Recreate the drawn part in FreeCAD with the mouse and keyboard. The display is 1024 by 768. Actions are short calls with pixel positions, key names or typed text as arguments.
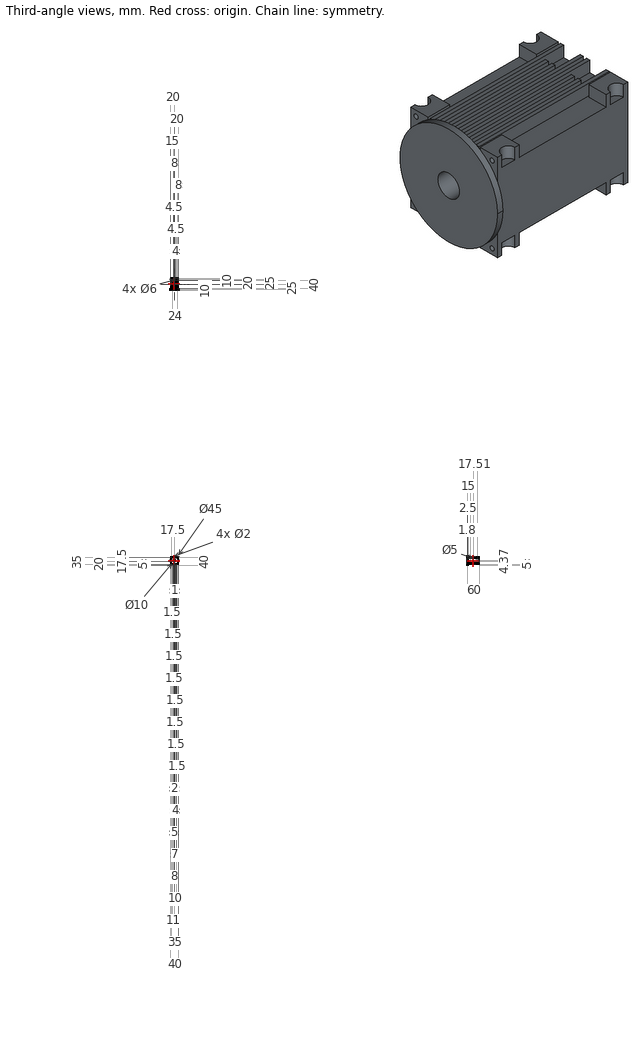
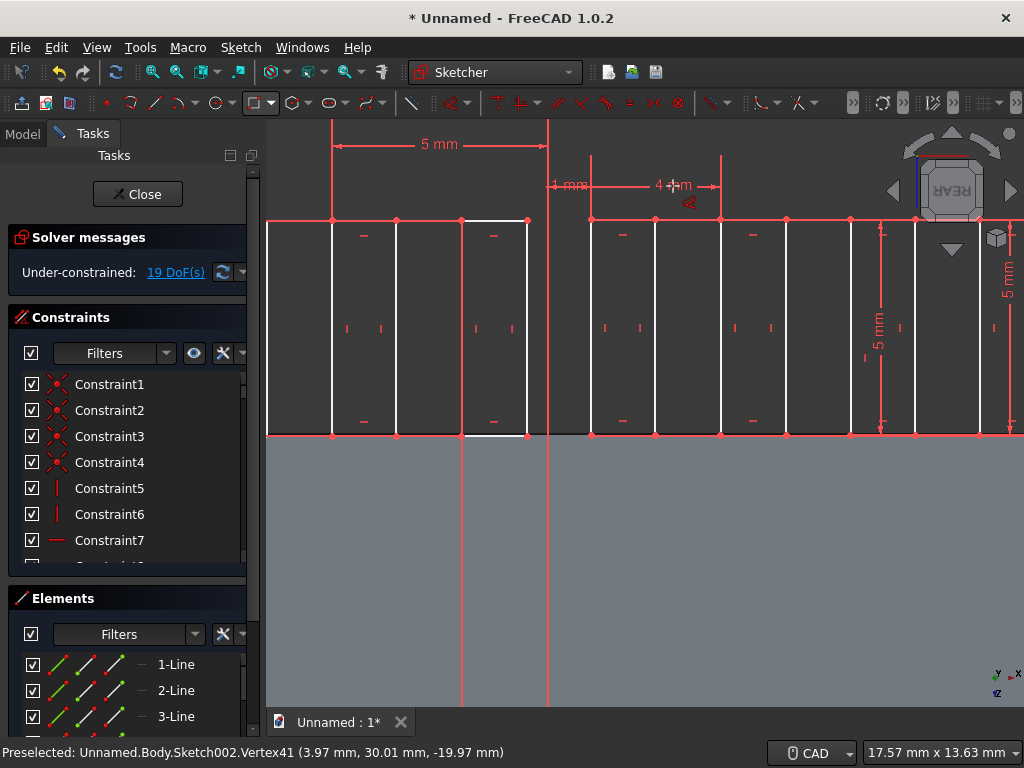
click(851, 220)
click(769, 186)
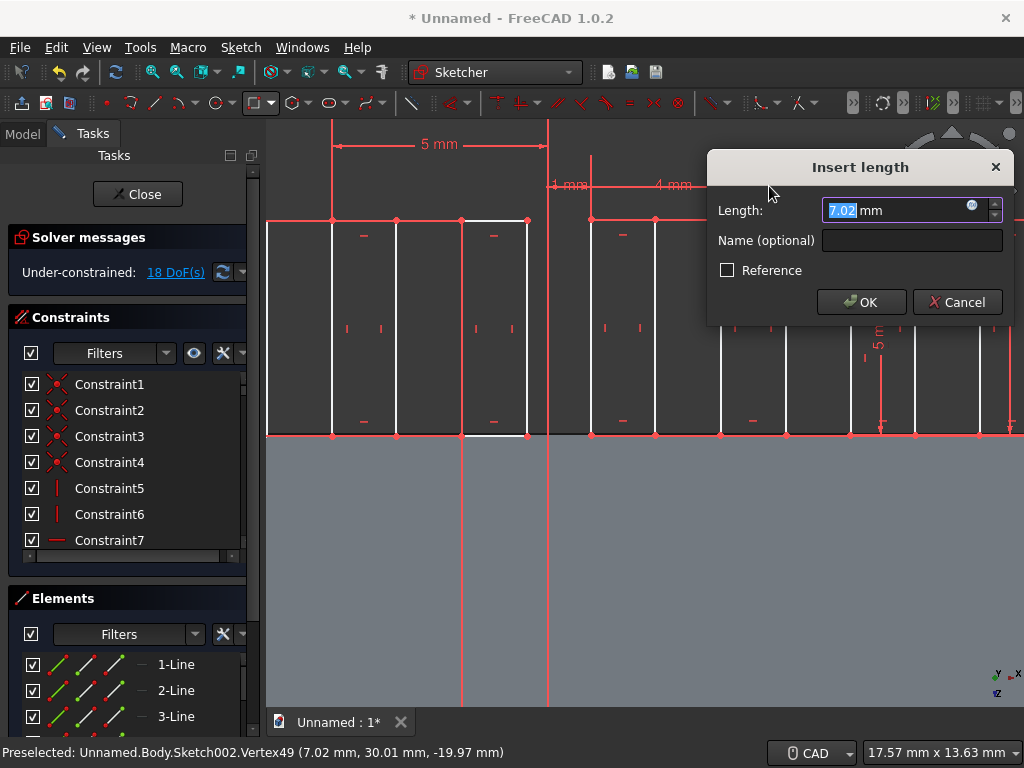
text(7)
key(Return)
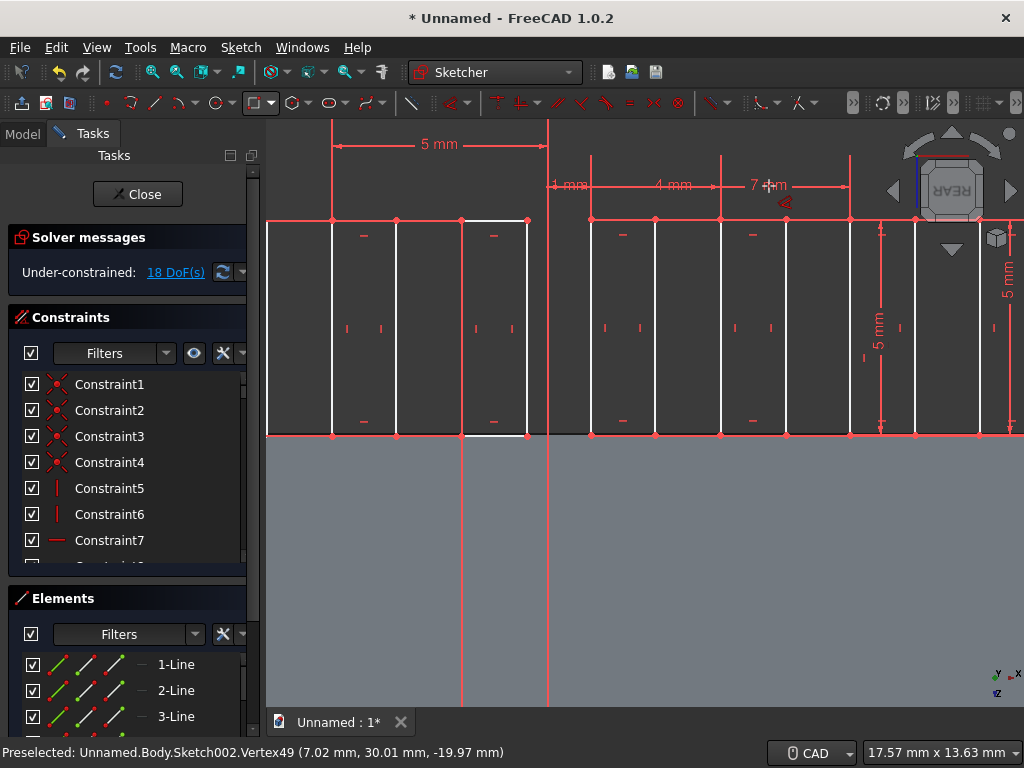
scroll(591, 220, down, 4)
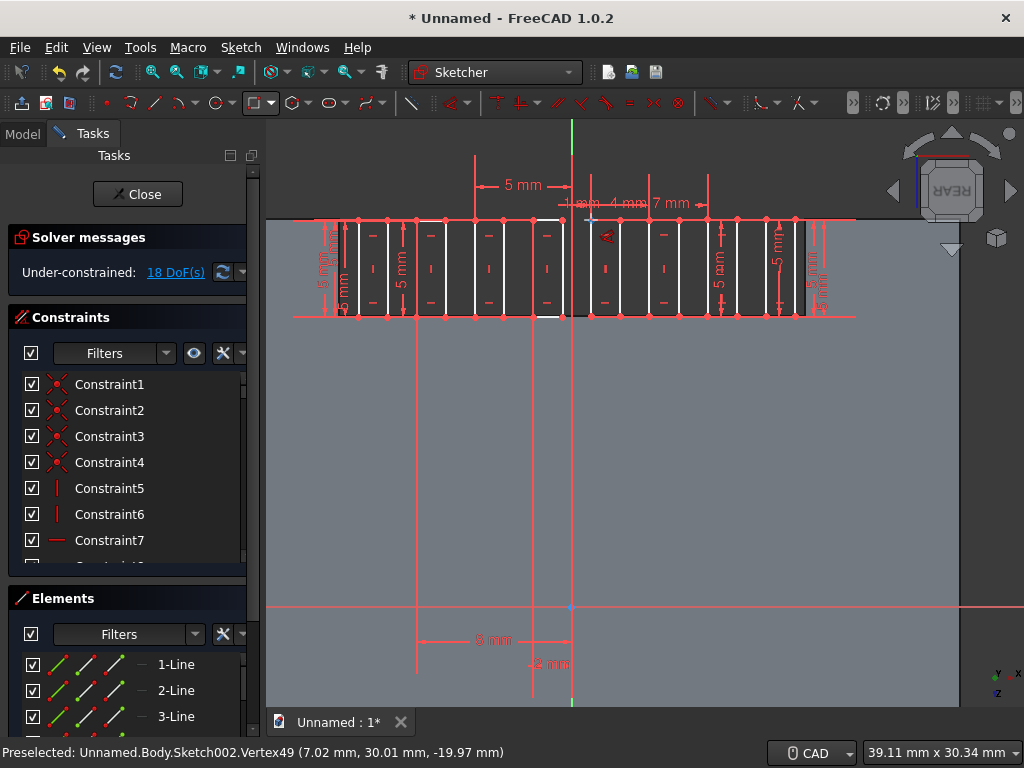
scroll(368, 317, up, 3)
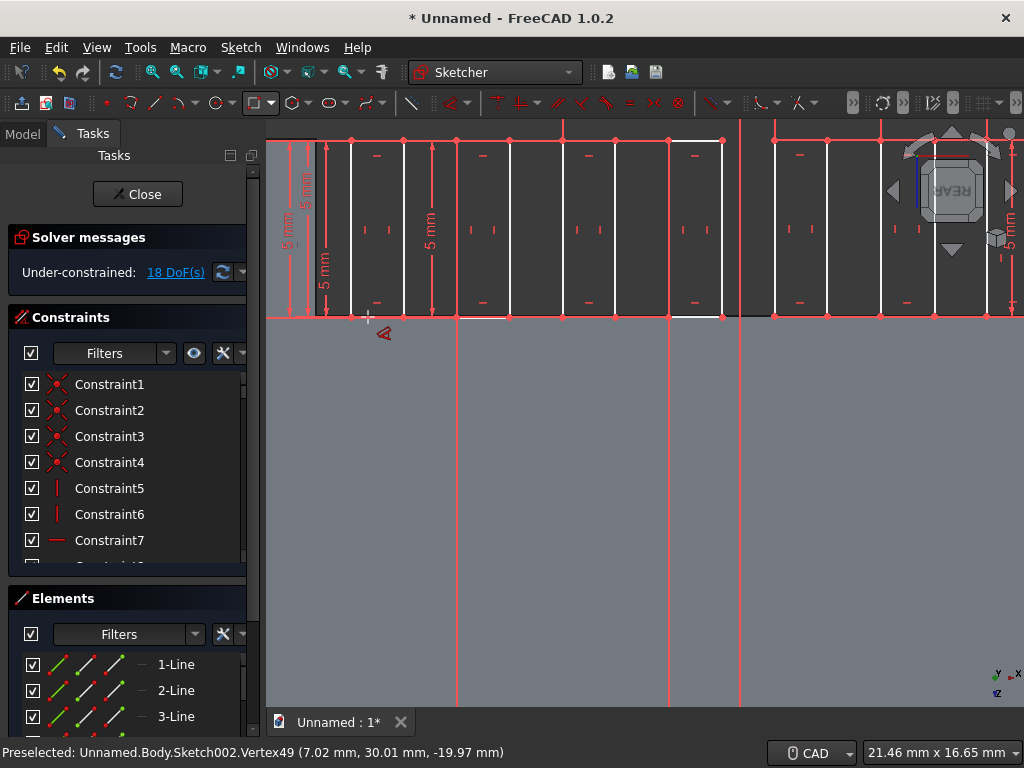
click(367, 318)
click(378, 352)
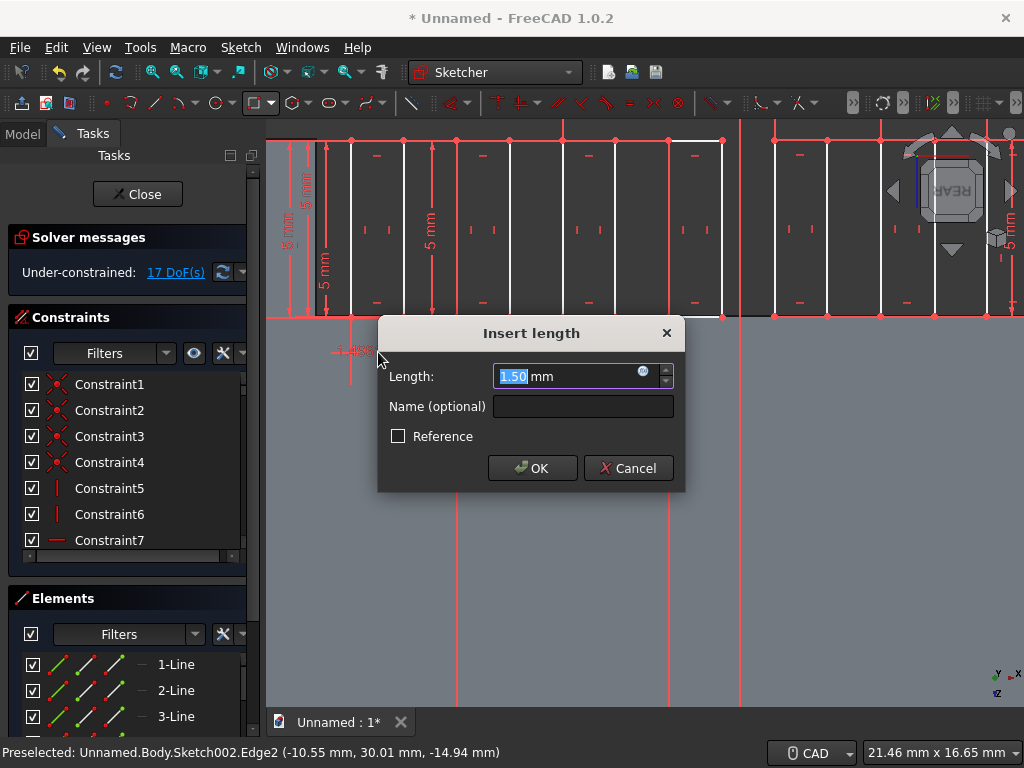
text(1.5)
key(Return)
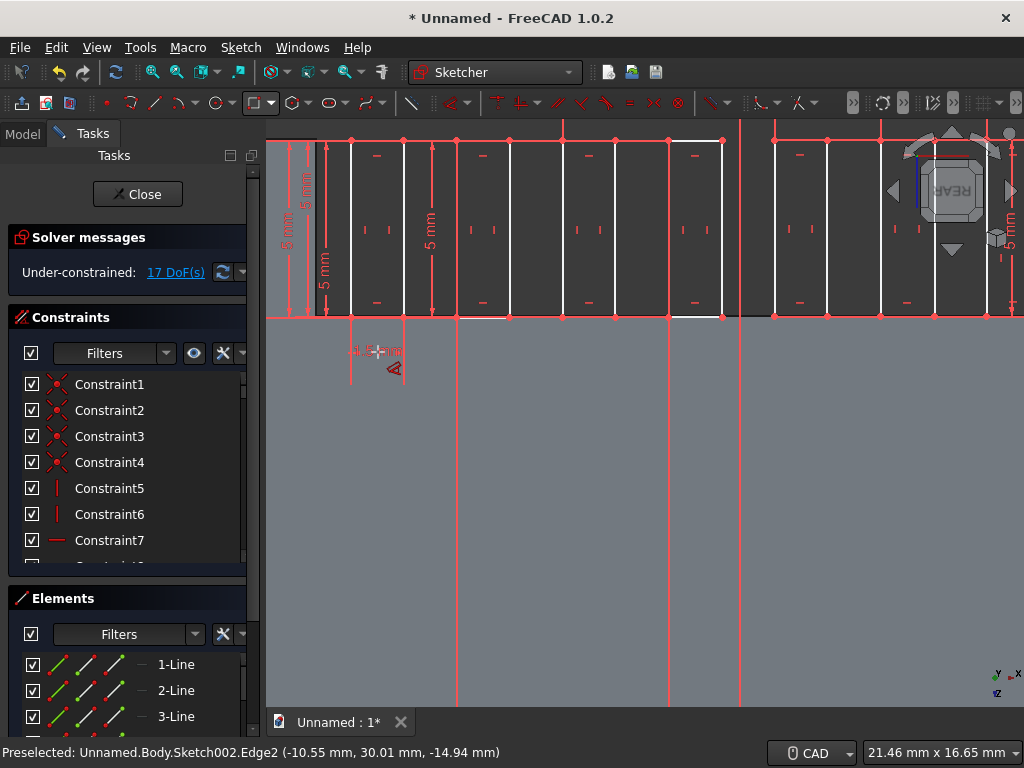
click(473, 318)
click(483, 284)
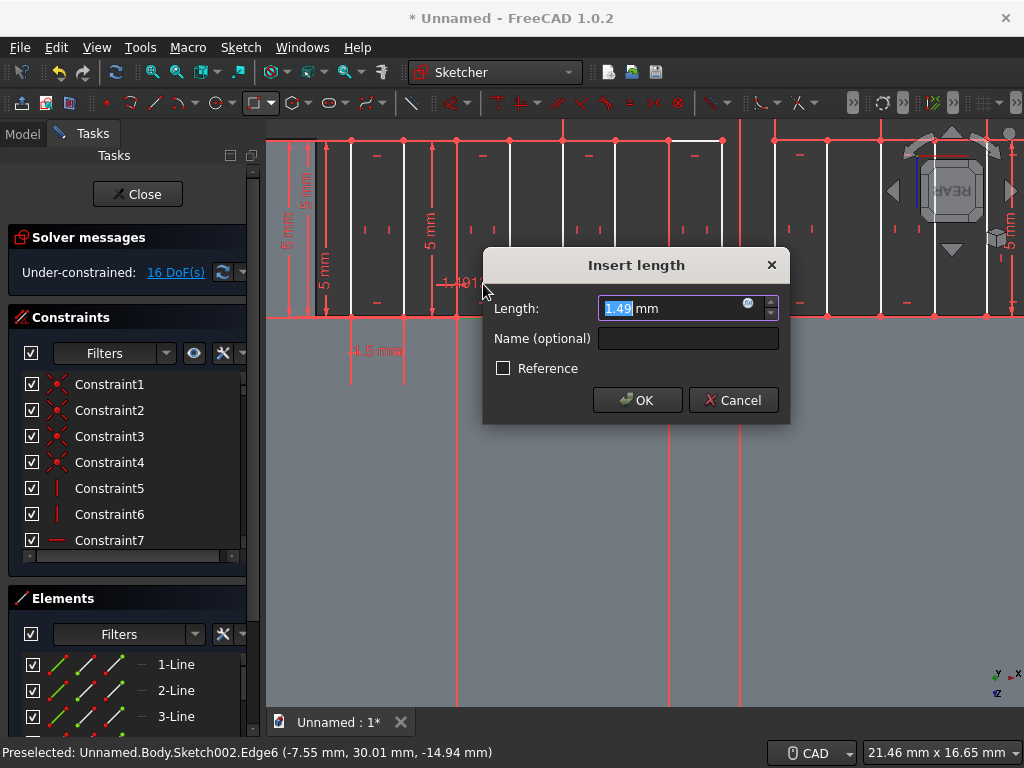
text(1.5)
key(Return)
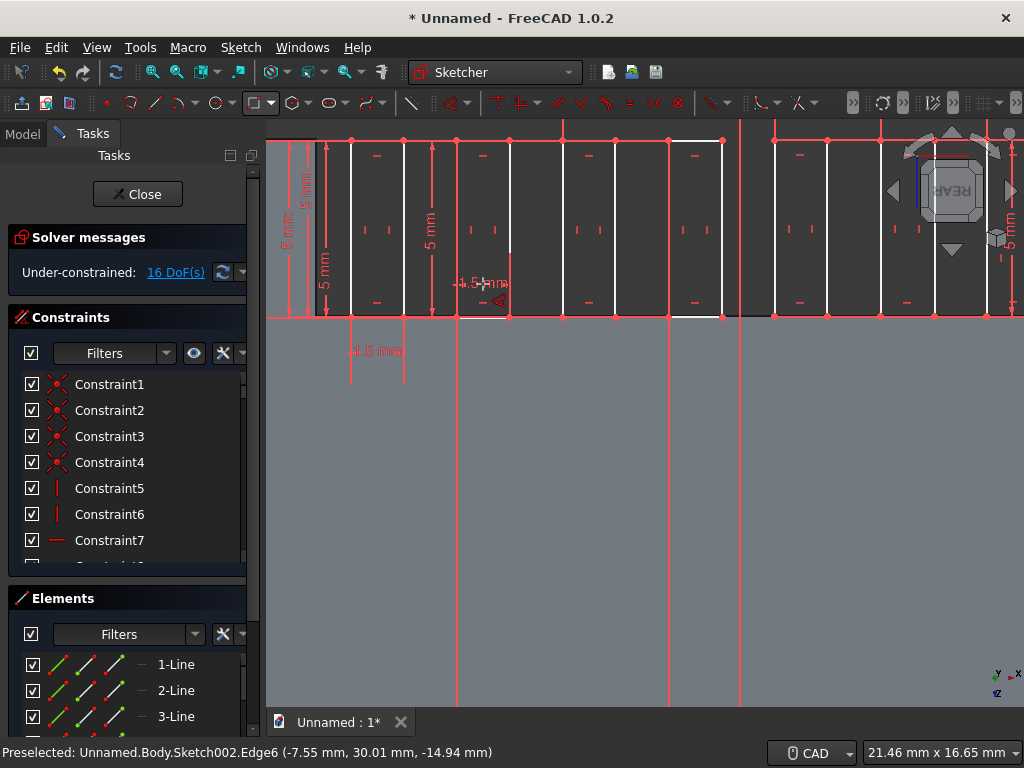
click(579, 317)
click(589, 283)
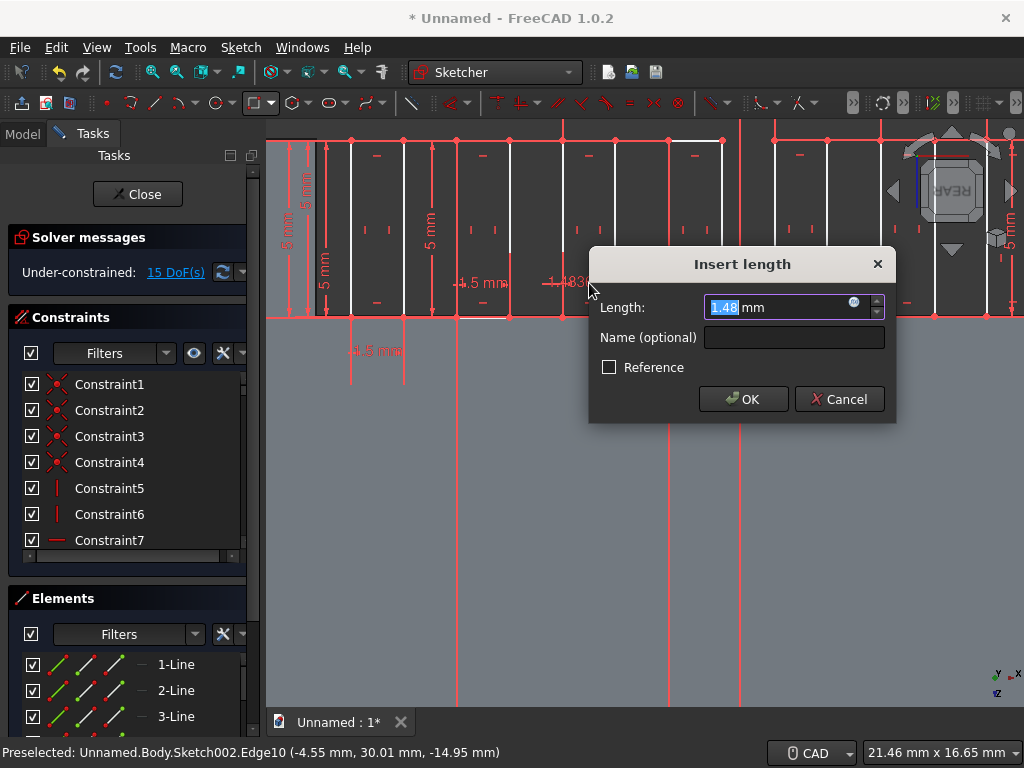
text(1.5)
key(Return)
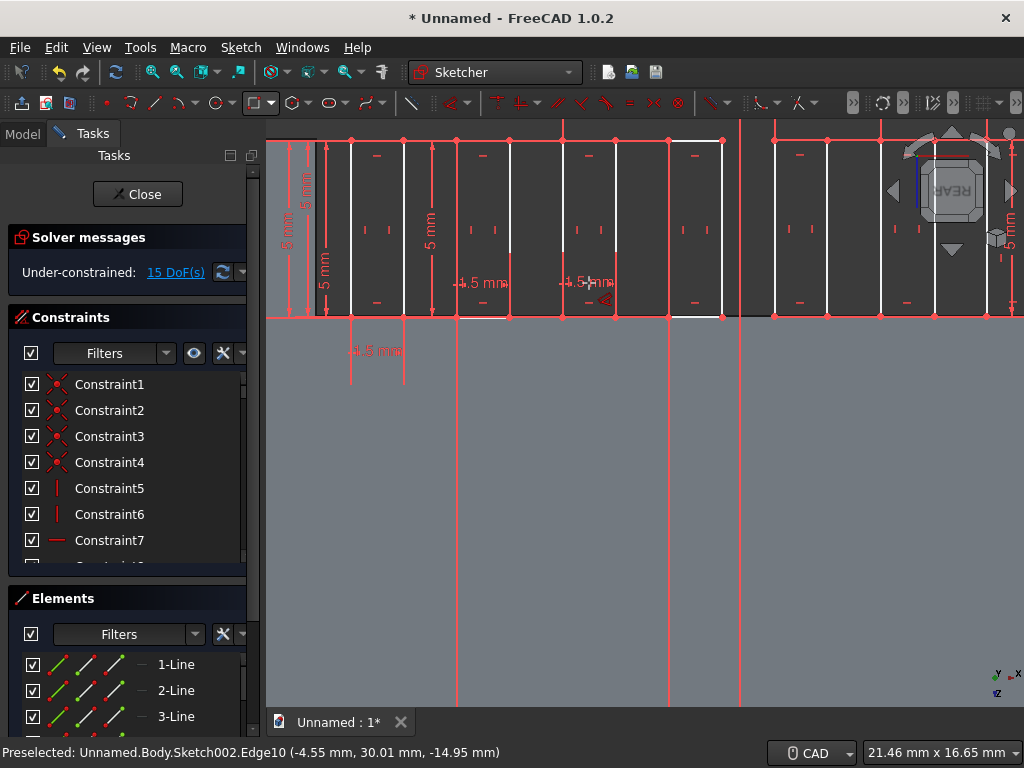
click(685, 317)
click(696, 283)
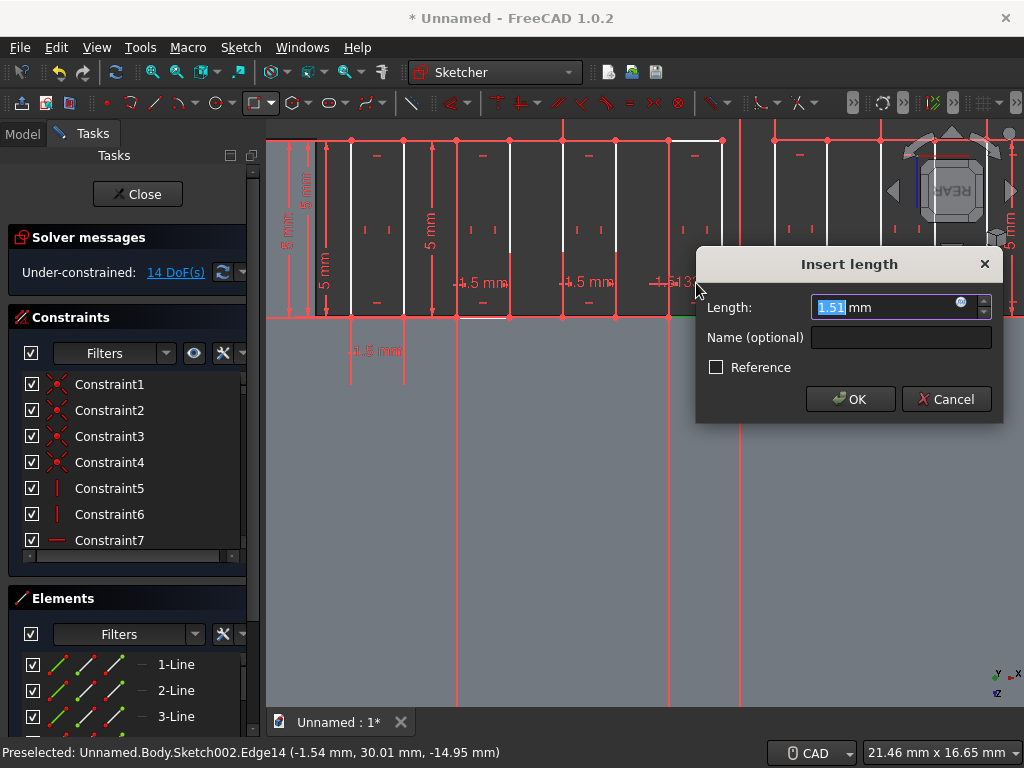
text(1.5)
key(Return)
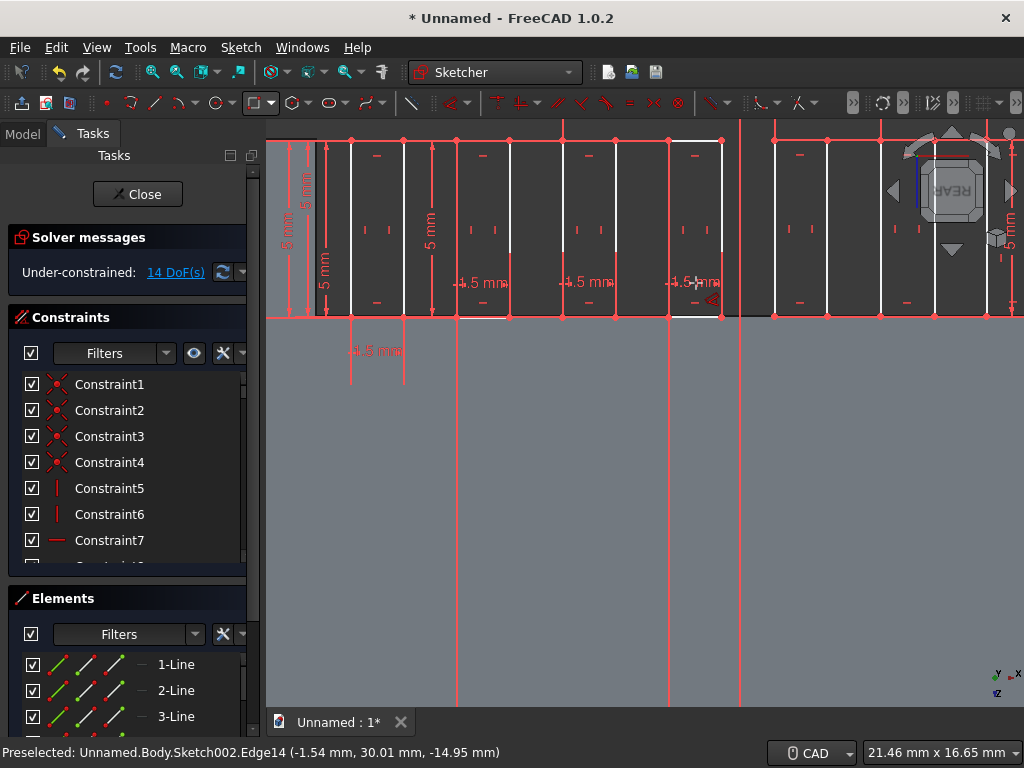
click(791, 317)
click(801, 283)